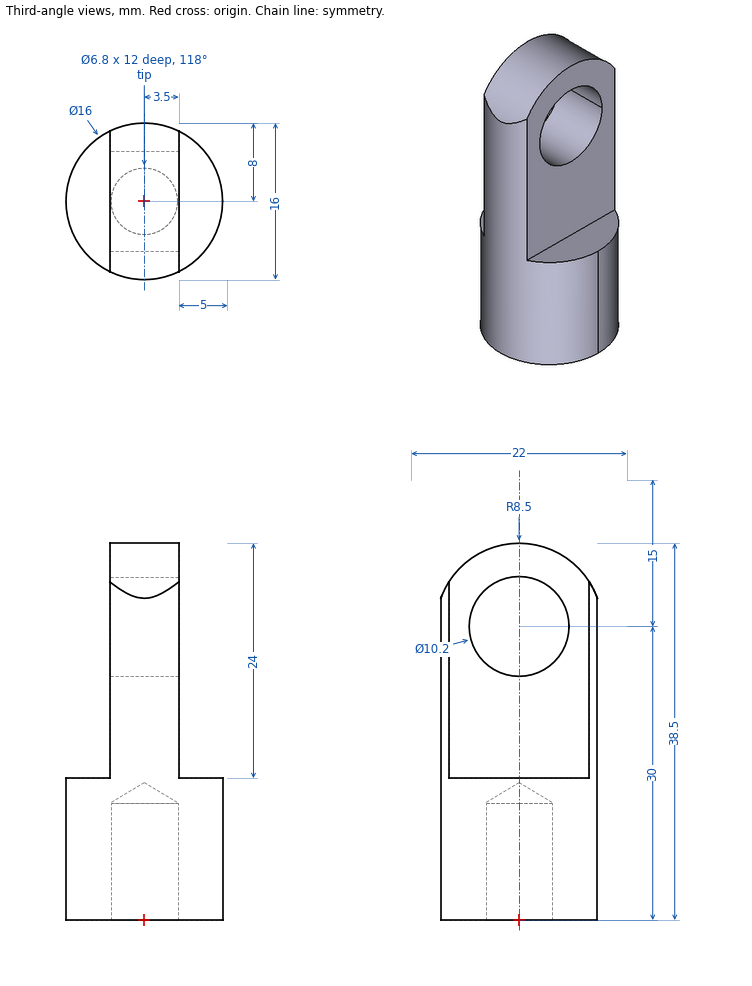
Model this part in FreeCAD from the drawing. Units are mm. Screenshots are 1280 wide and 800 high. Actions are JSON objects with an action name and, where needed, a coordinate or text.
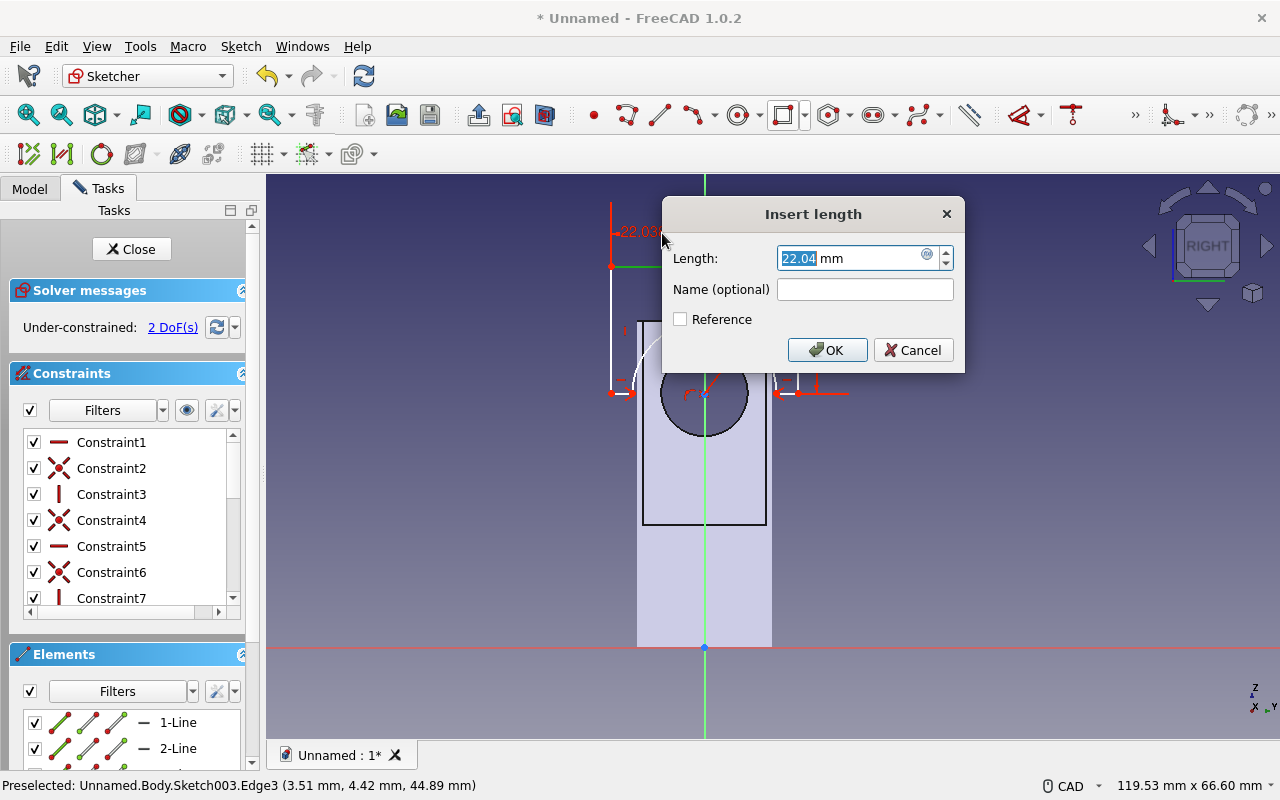
{"action": "type", "text": "22"}
{"action": "key", "text": "Return"}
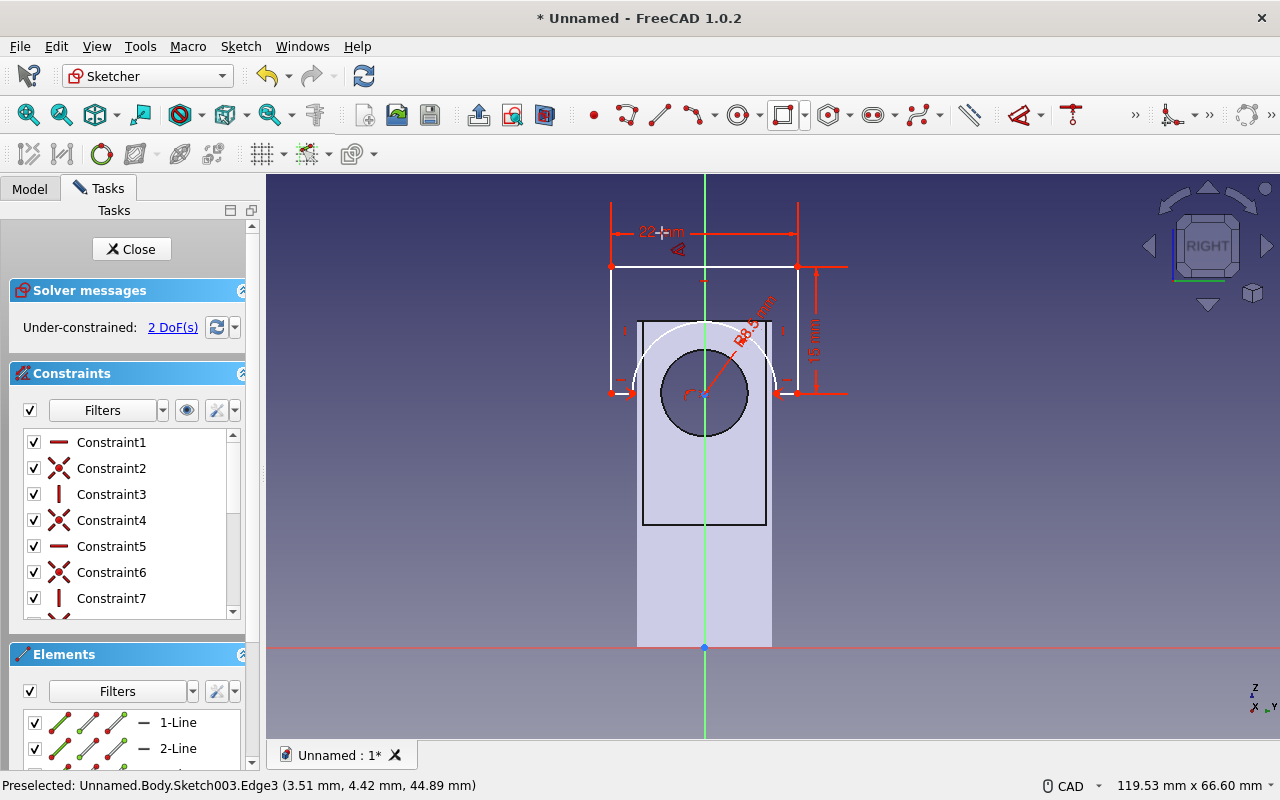
{"action": "left_click", "coordinate": [777, 394]}
{"action": "left_click", "coordinate": [811, 521]}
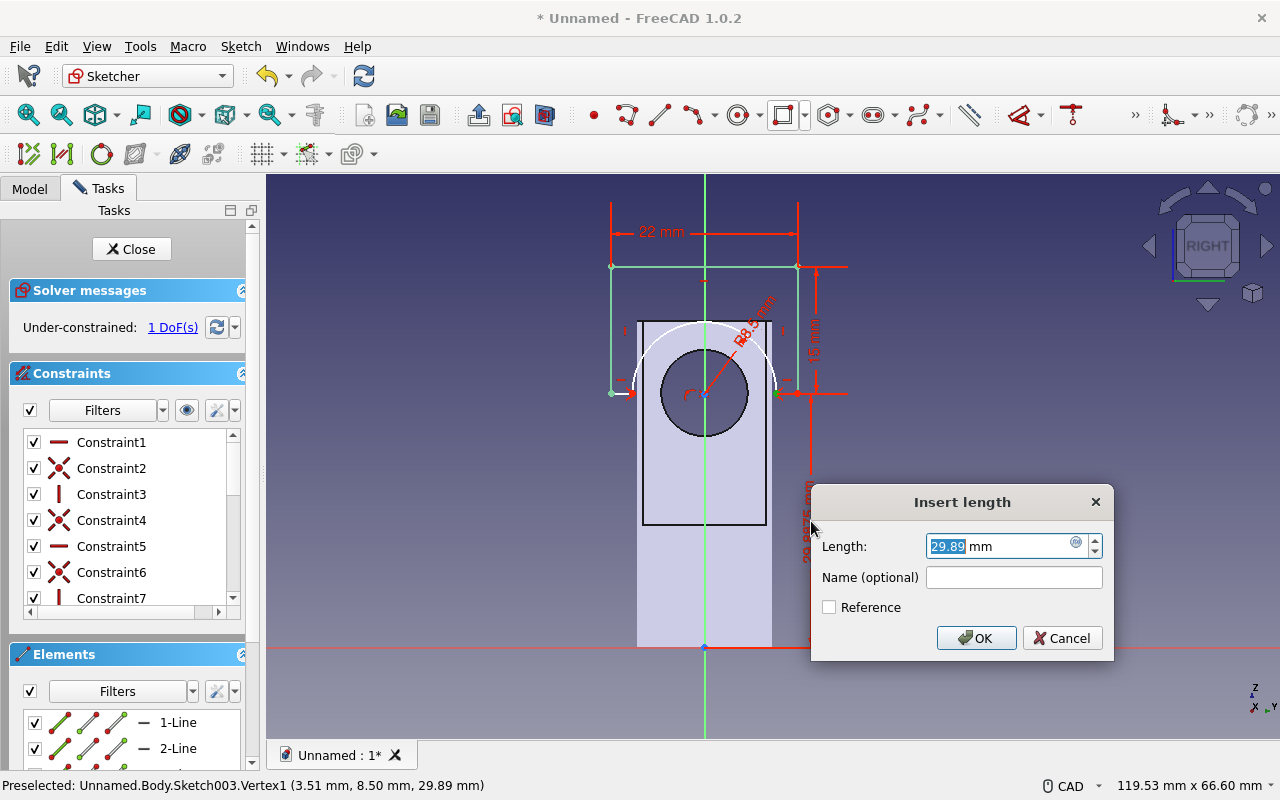
{"action": "type", "text": "30"}
{"action": "key", "text": "Return"}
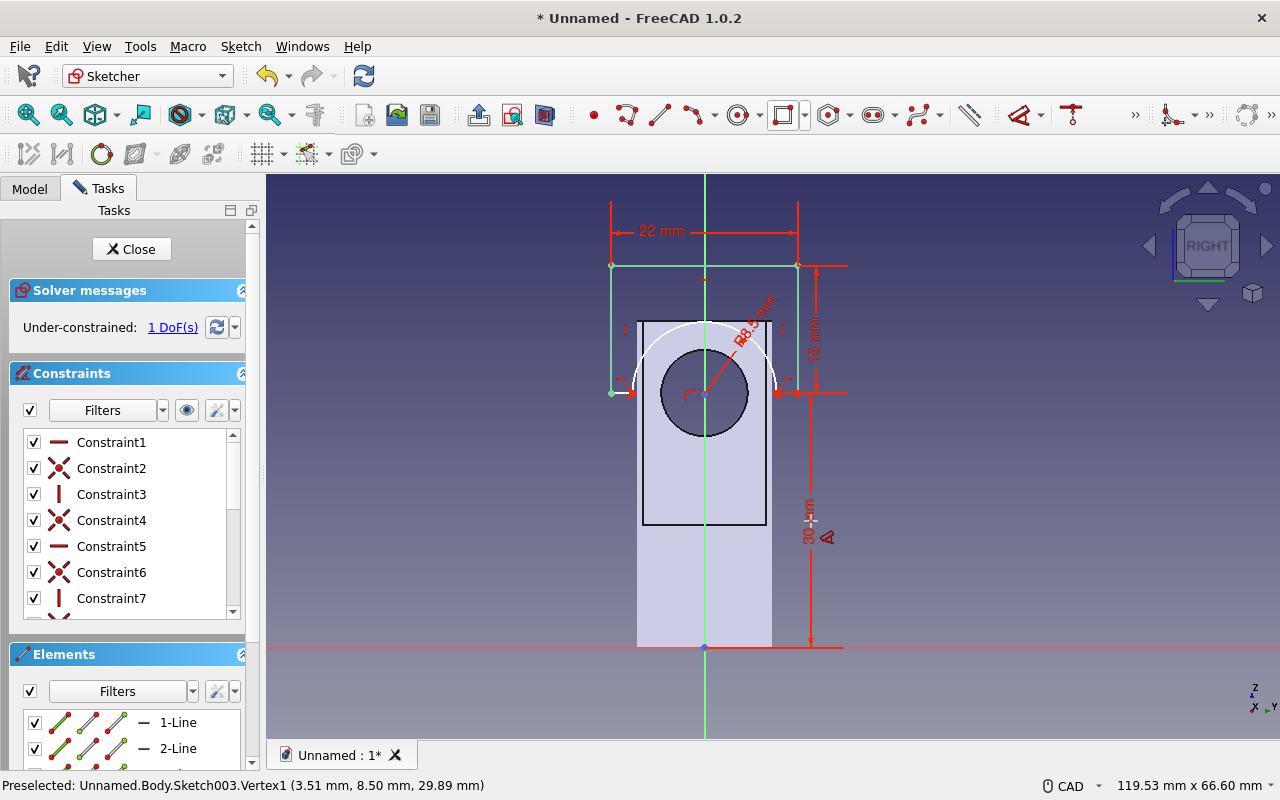
{"action": "left_click", "coordinate": [705, 394]}
{"action": "left_click", "coordinate": [739, 521]}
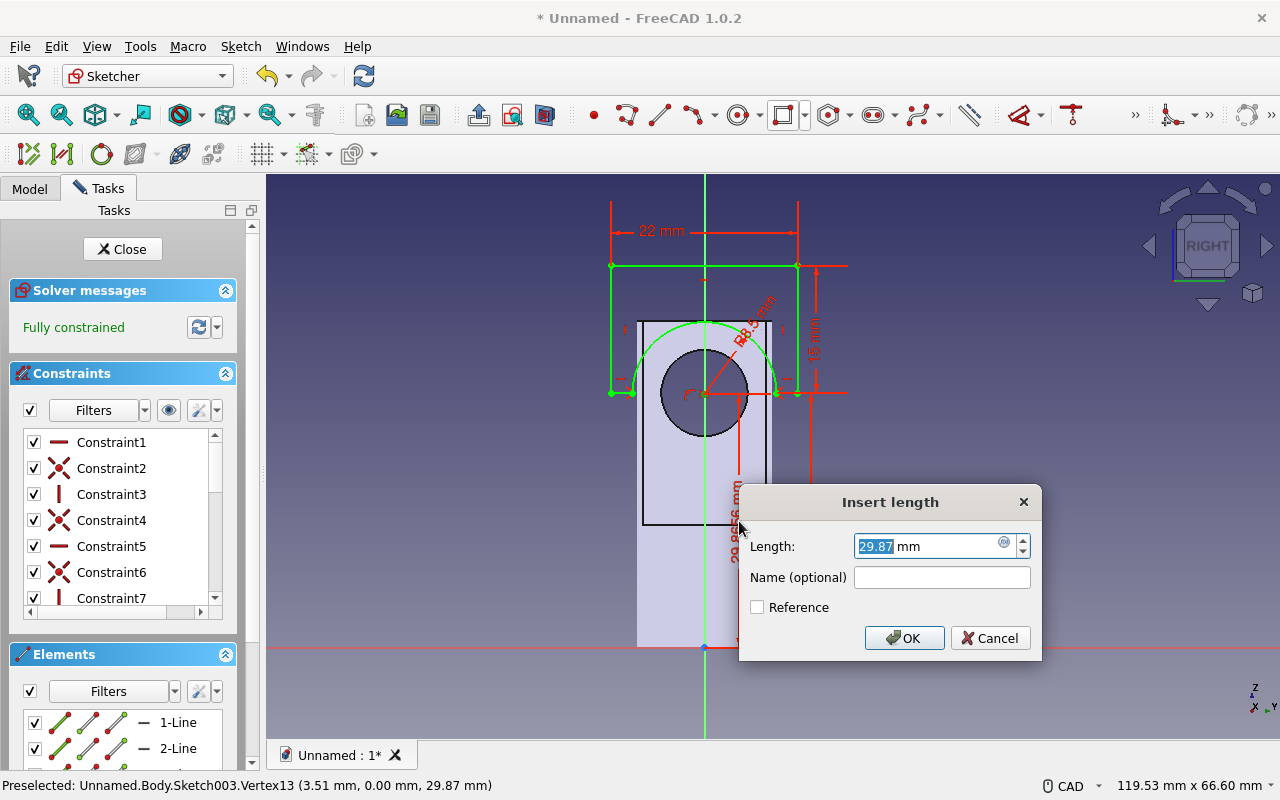
{"action": "type", "text": "30"}
{"action": "key", "text": "Return"}
{"action": "key", "text": "Escape"}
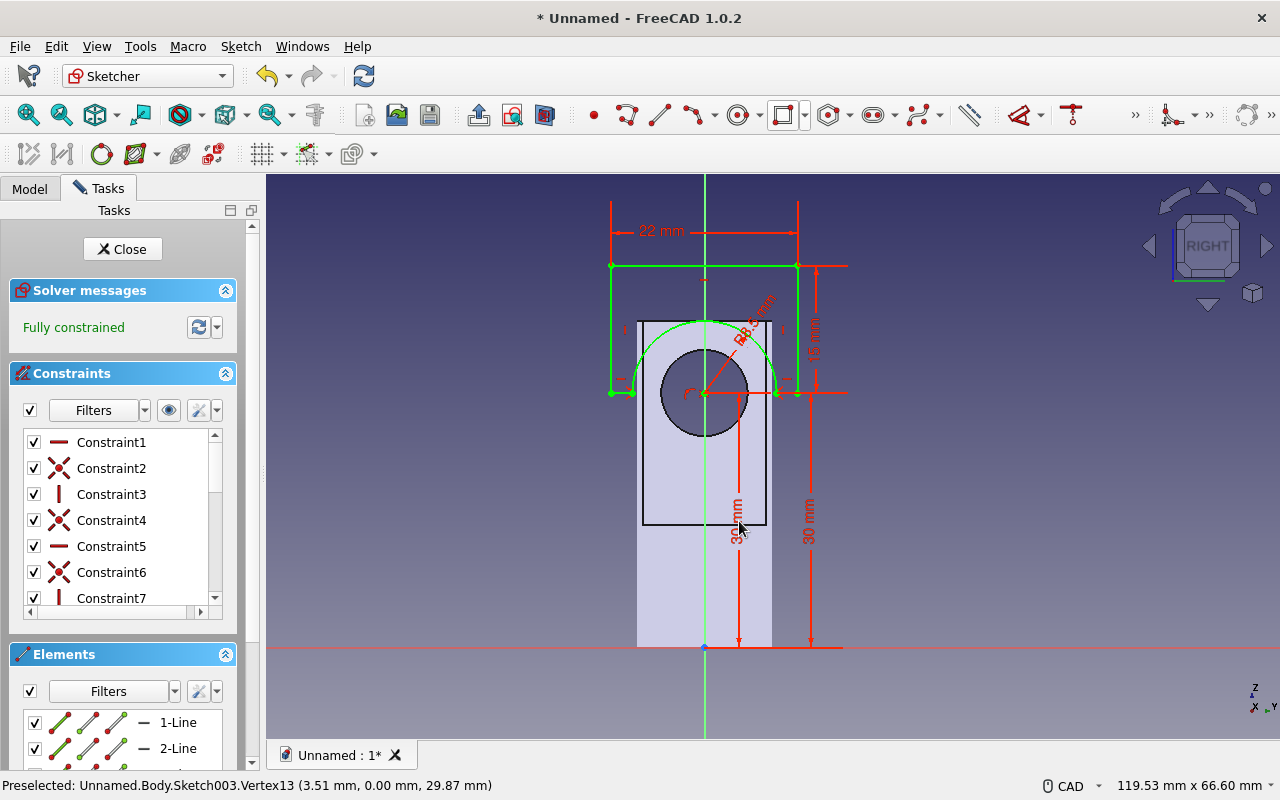
{"action": "left_click", "coordinate": [123, 249]}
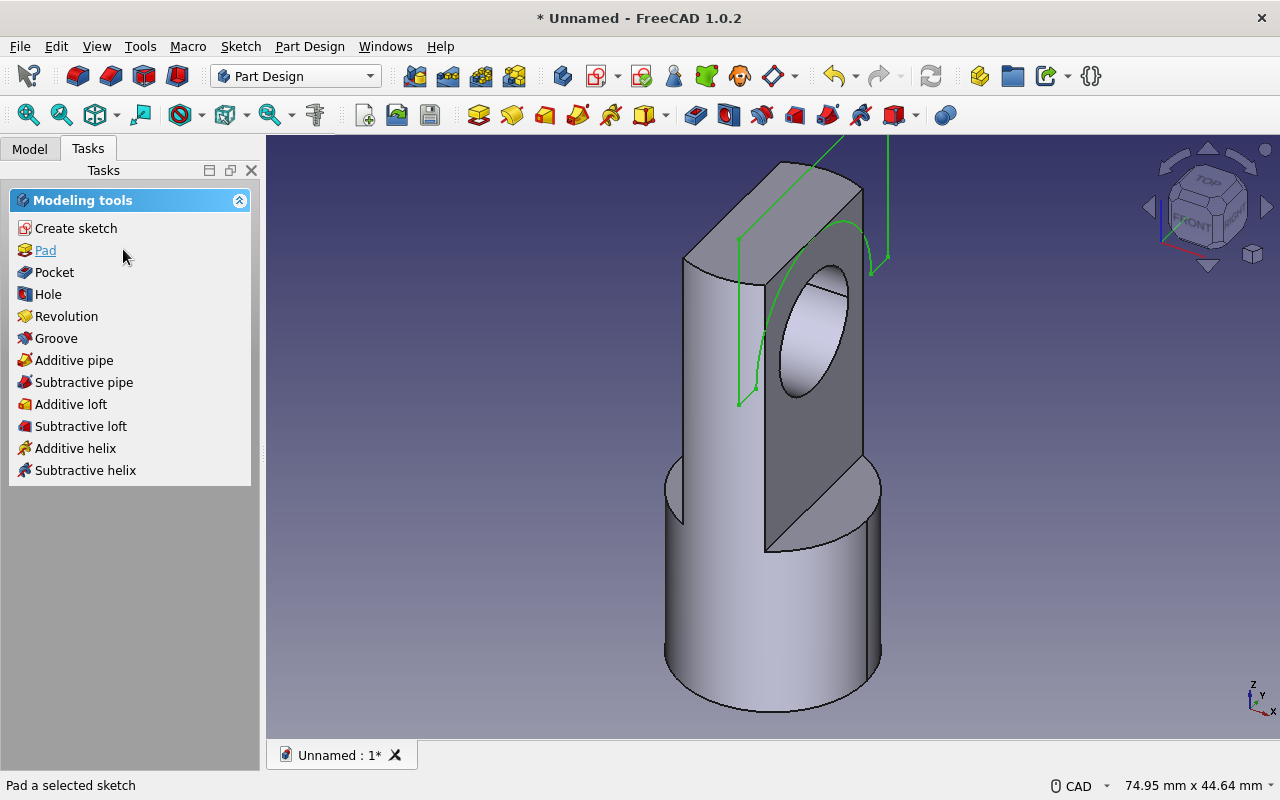
{"action": "left_click", "coordinate": [696, 116]}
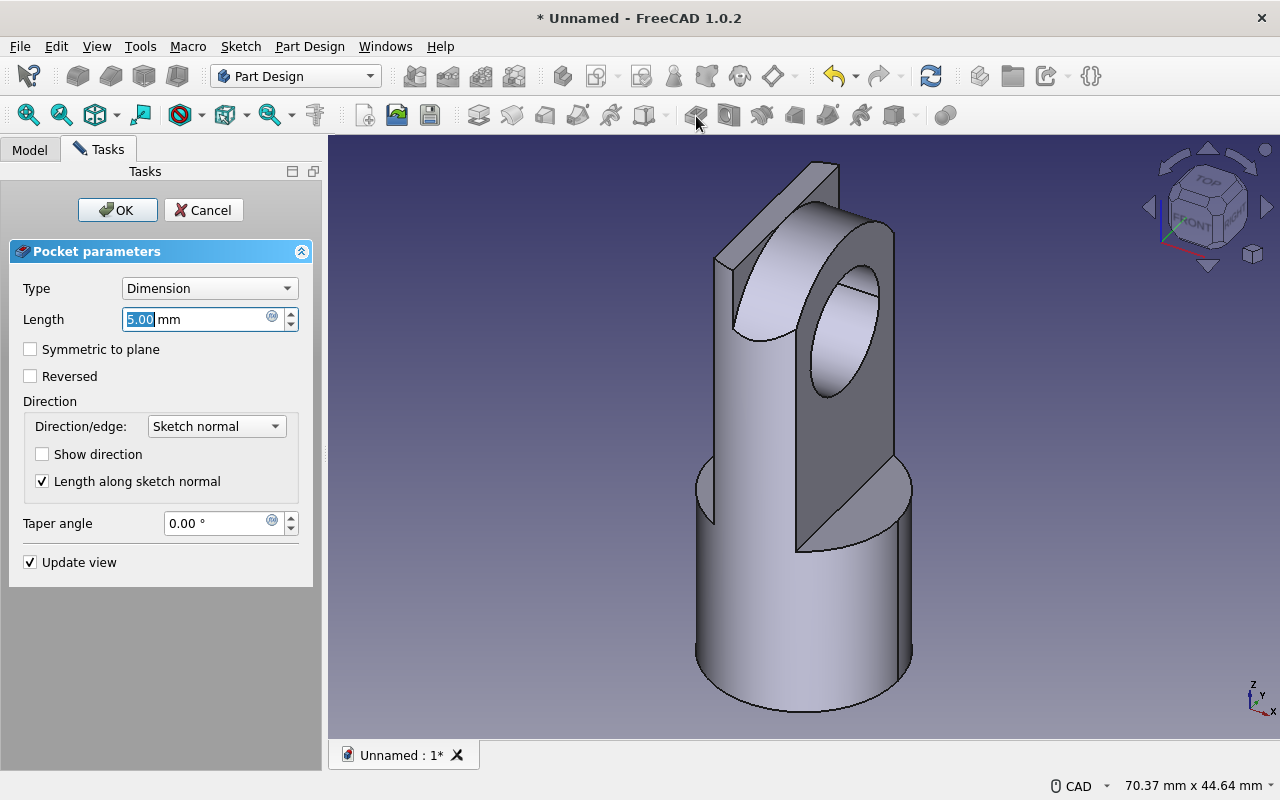
{"action": "left_click", "coordinate": [210, 288]}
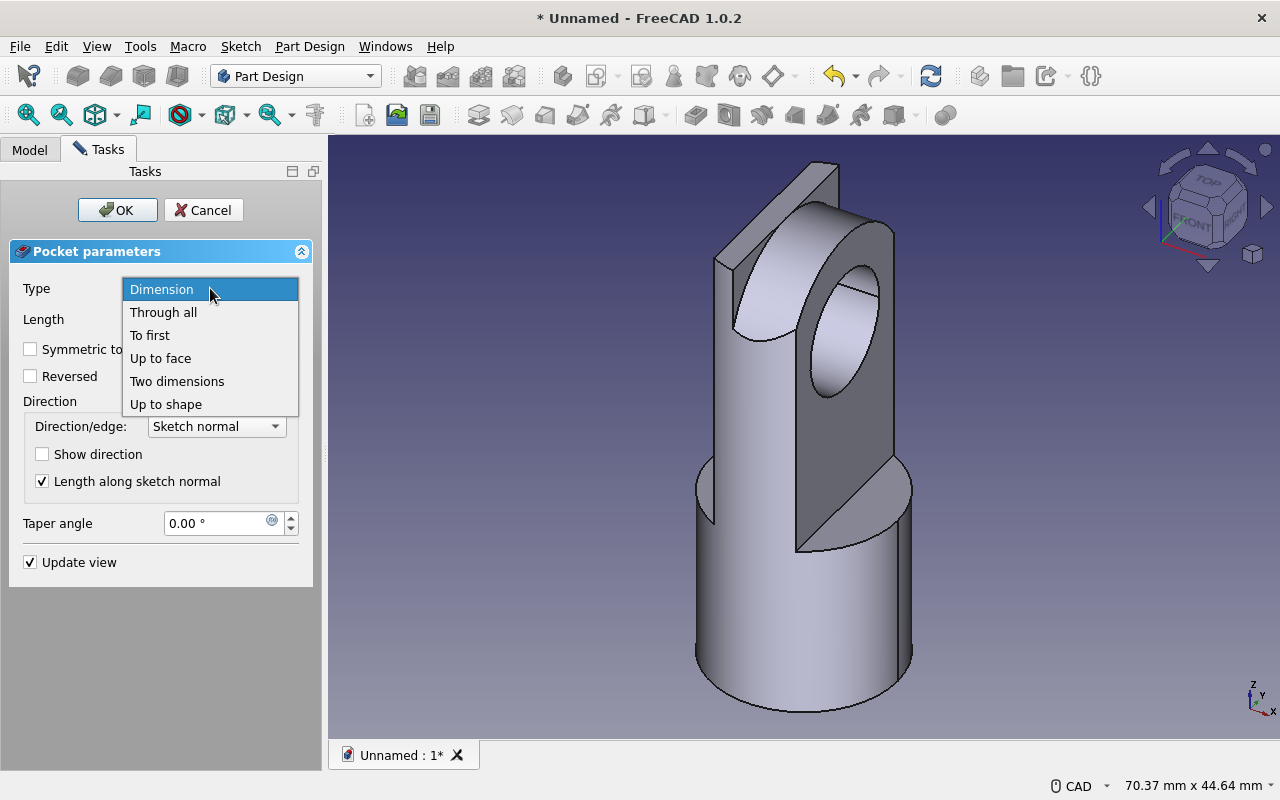
{"action": "left_click", "coordinate": [208, 312]}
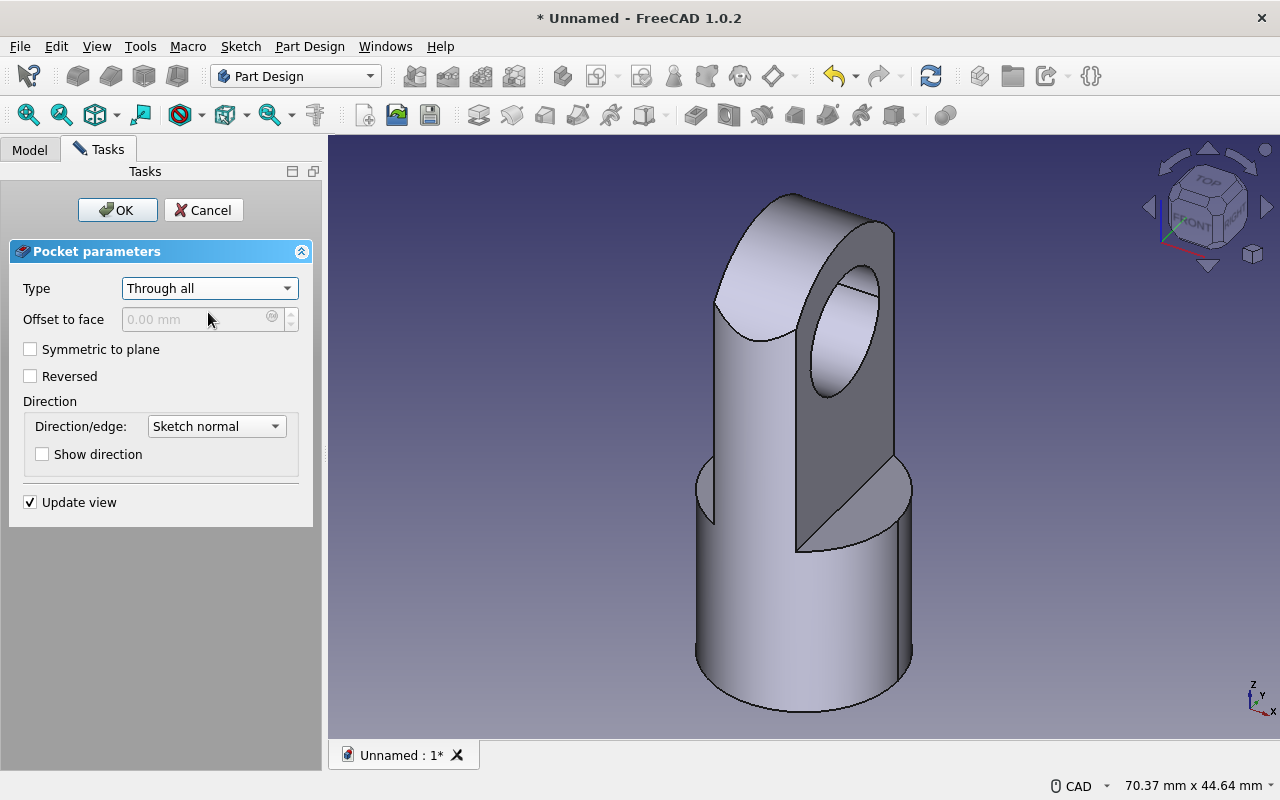
{"action": "left_click", "coordinate": [118, 210]}